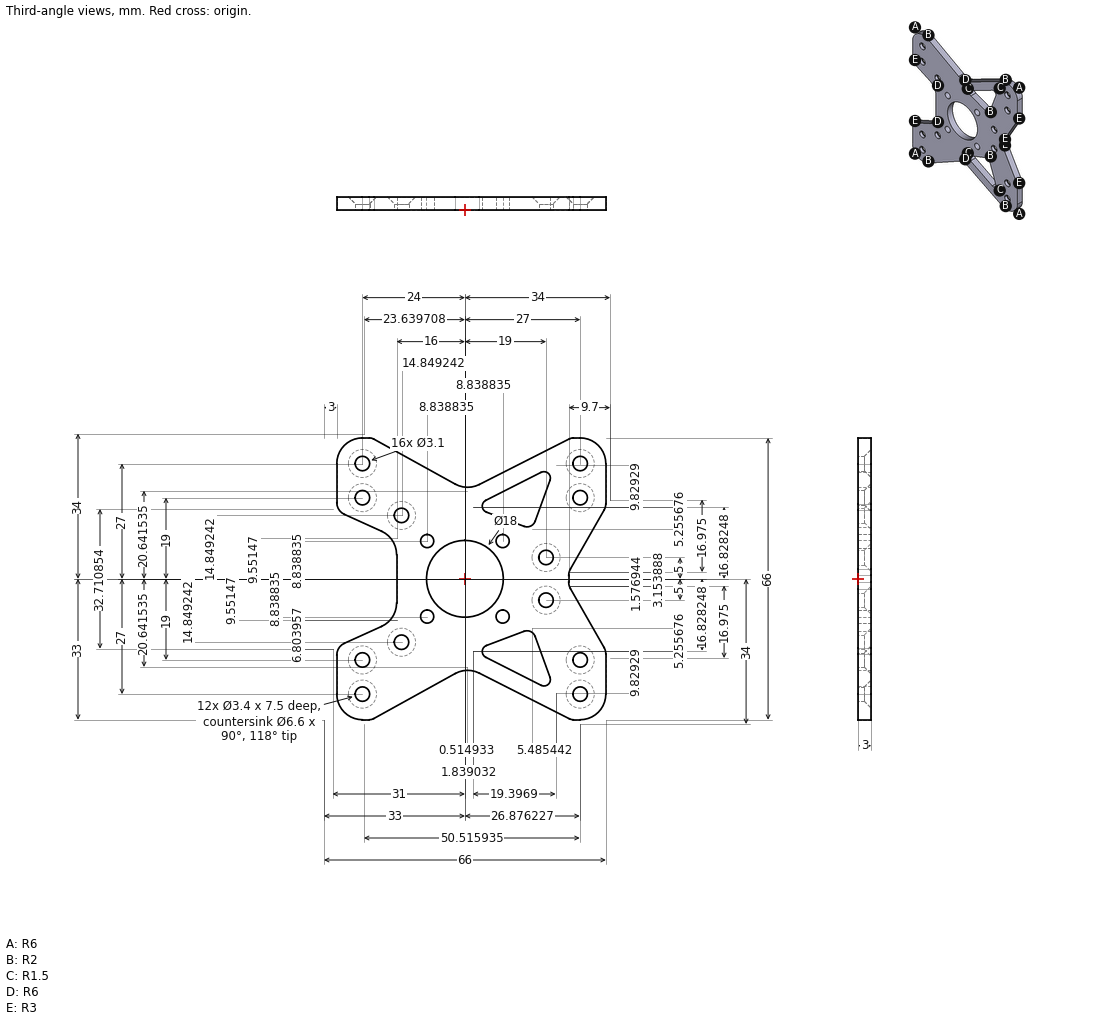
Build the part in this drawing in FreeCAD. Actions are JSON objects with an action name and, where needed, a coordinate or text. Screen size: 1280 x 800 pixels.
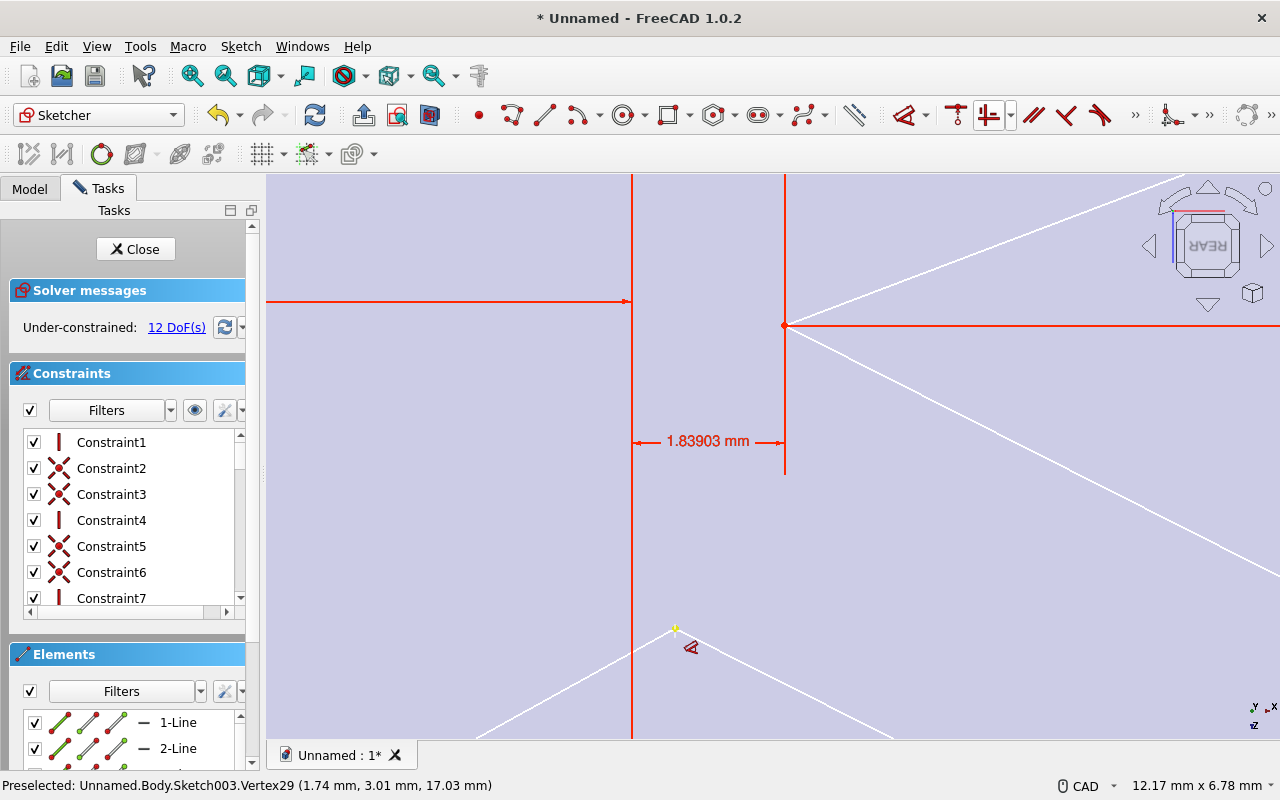
{"action": "left_click", "coordinate": [675, 629]}
{"action": "left_click", "coordinate": [653, 663]}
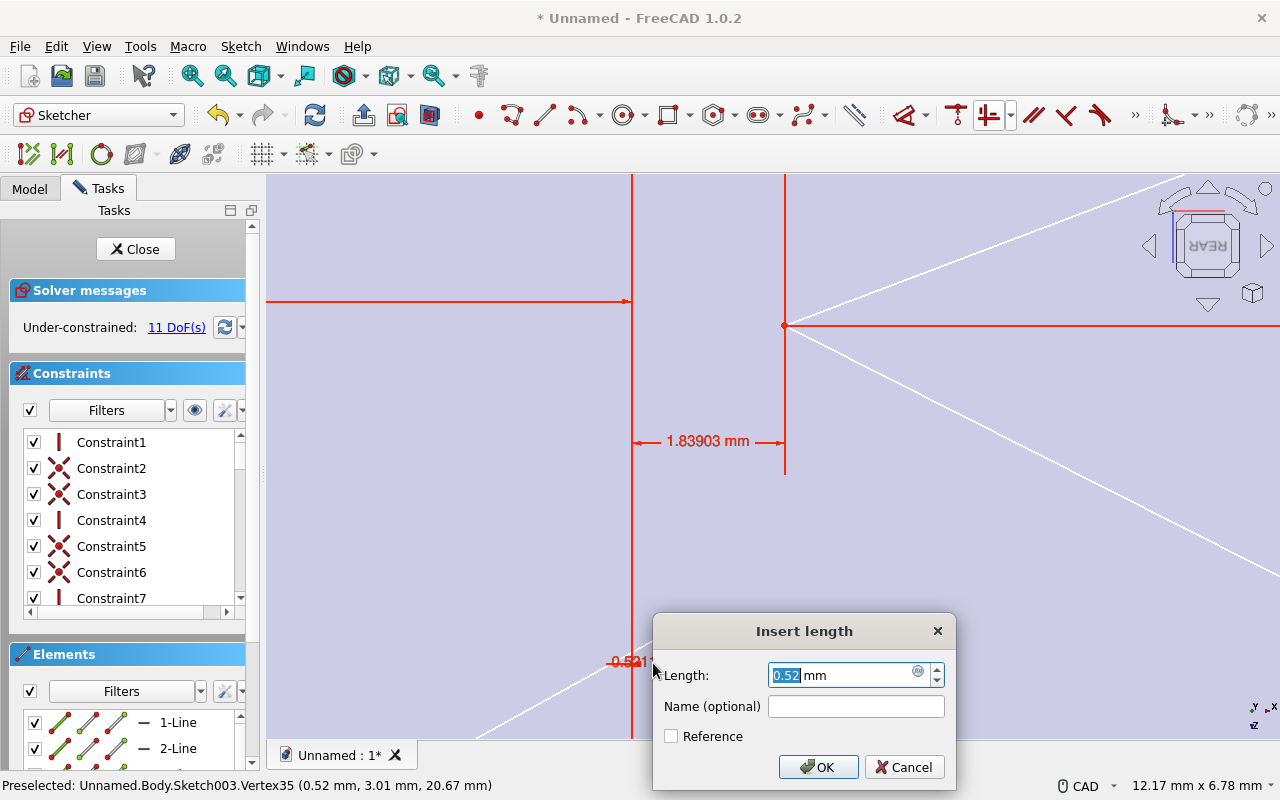
{"action": "type", "text": "0.514933"}
{"action": "key", "text": "Return"}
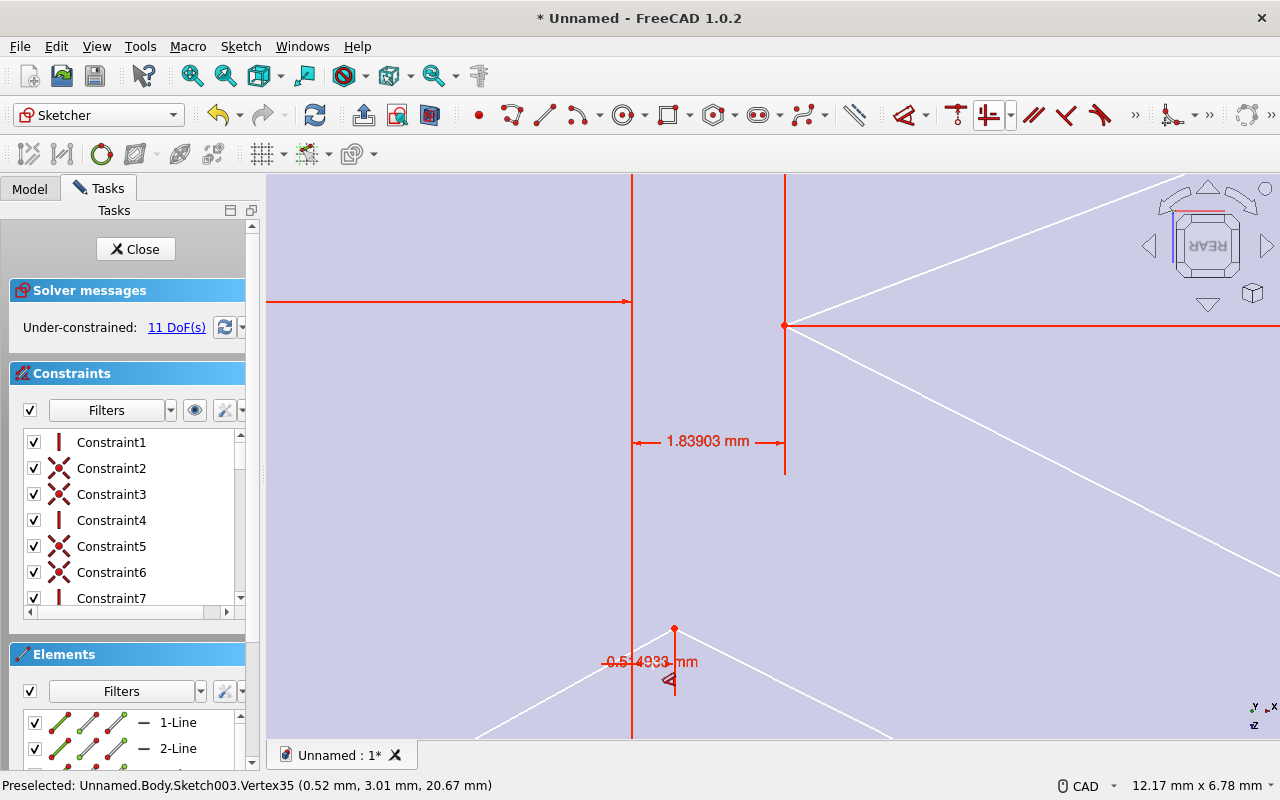
{"action": "scroll", "coordinate": [701, 557], "scroll_direction": "down", "scroll_amount": 14}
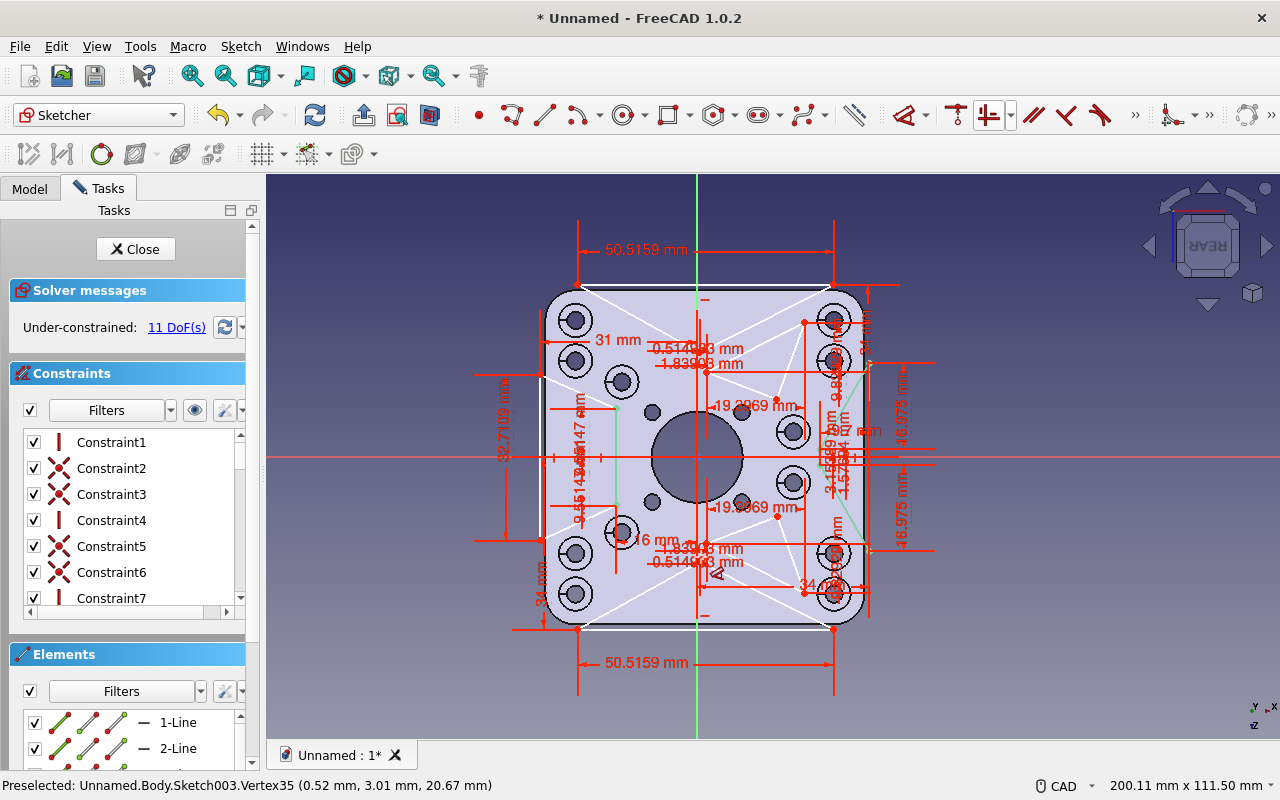
{"action": "left_click", "coordinate": [593, 399]}
{"action": "left_click", "coordinate": [506, 392]}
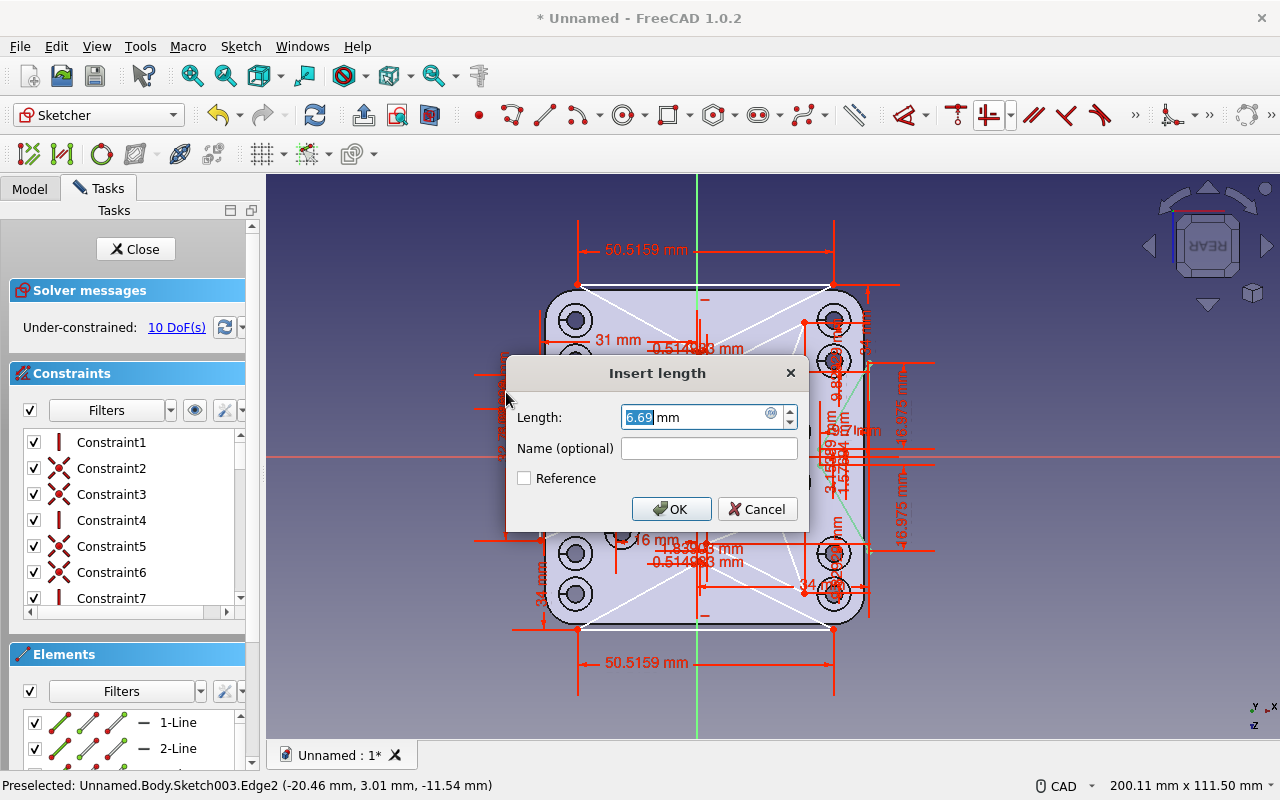
{"action": "type", "text": "6.803957"}
{"action": "key", "text": "Return"}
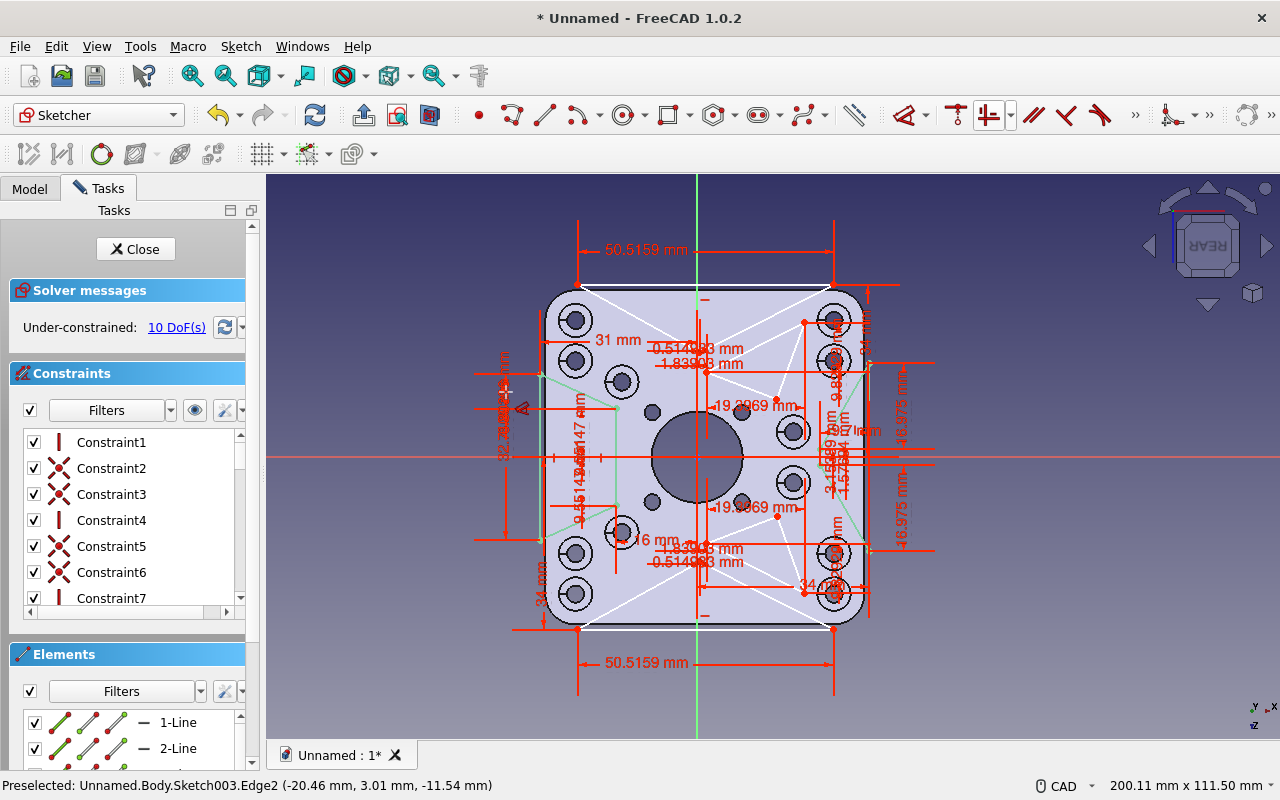
{"action": "scroll", "coordinate": [728, 380], "scroll_direction": "up", "scroll_amount": 2}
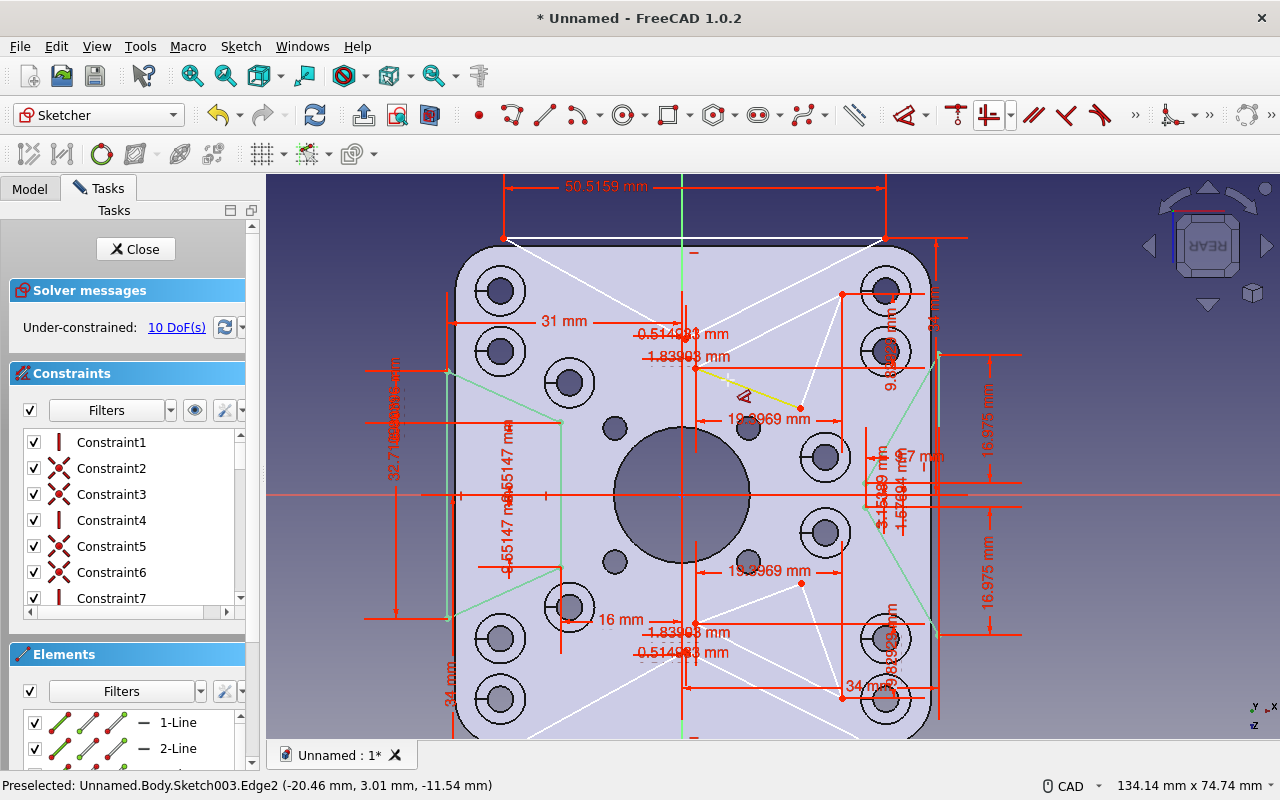
{"action": "left_click", "coordinate": [727, 380]}
{"action": "left_click", "coordinate": [835, 389]}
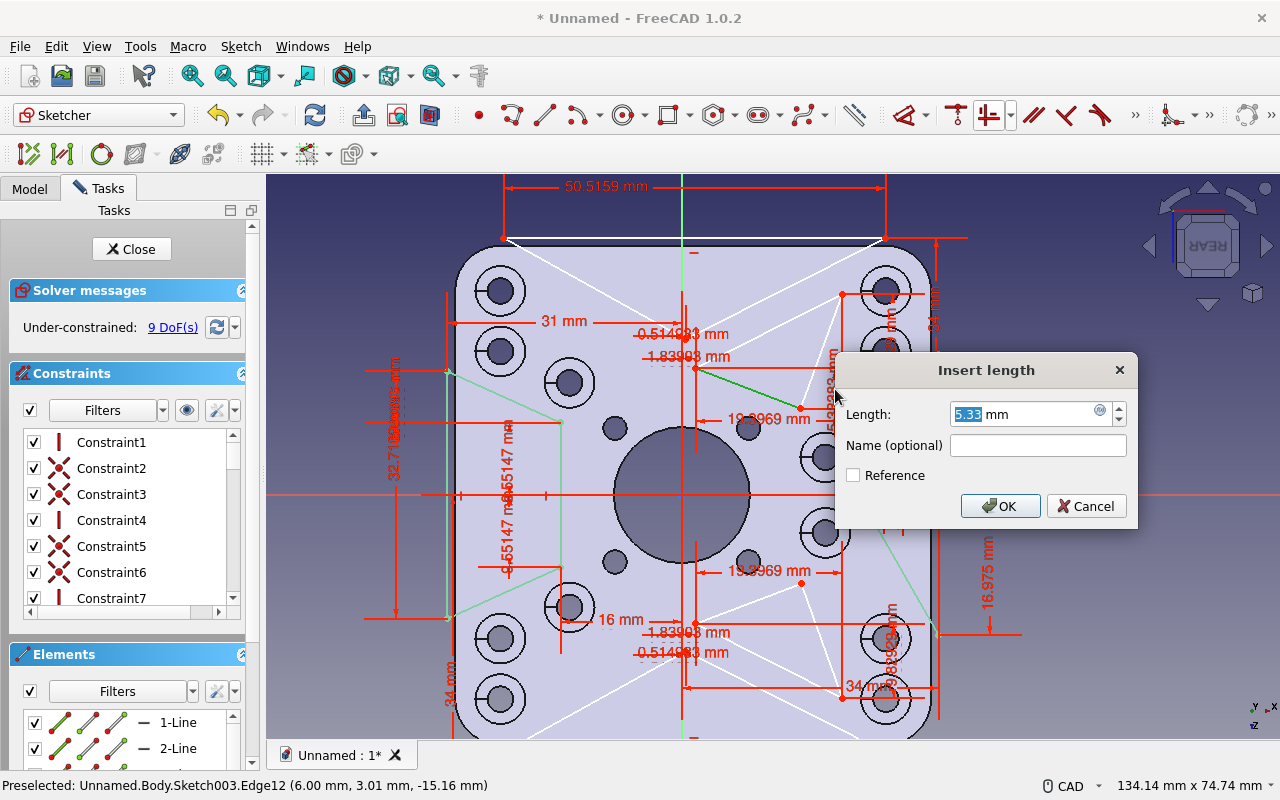
{"action": "type", "text": "5.255676"}
{"action": "key", "text": "Return"}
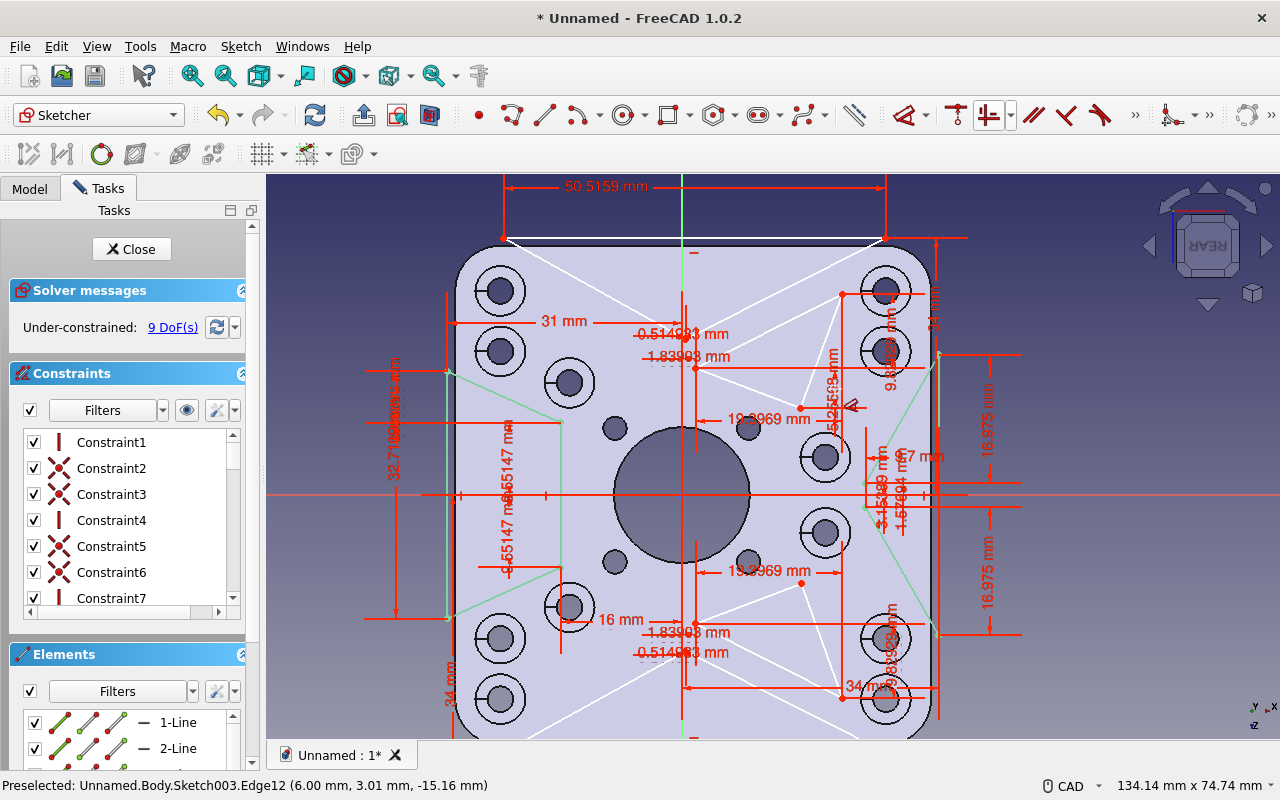
{"action": "left_click", "coordinate": [813, 374]}
{"action": "left_click", "coordinate": [812, 260]}